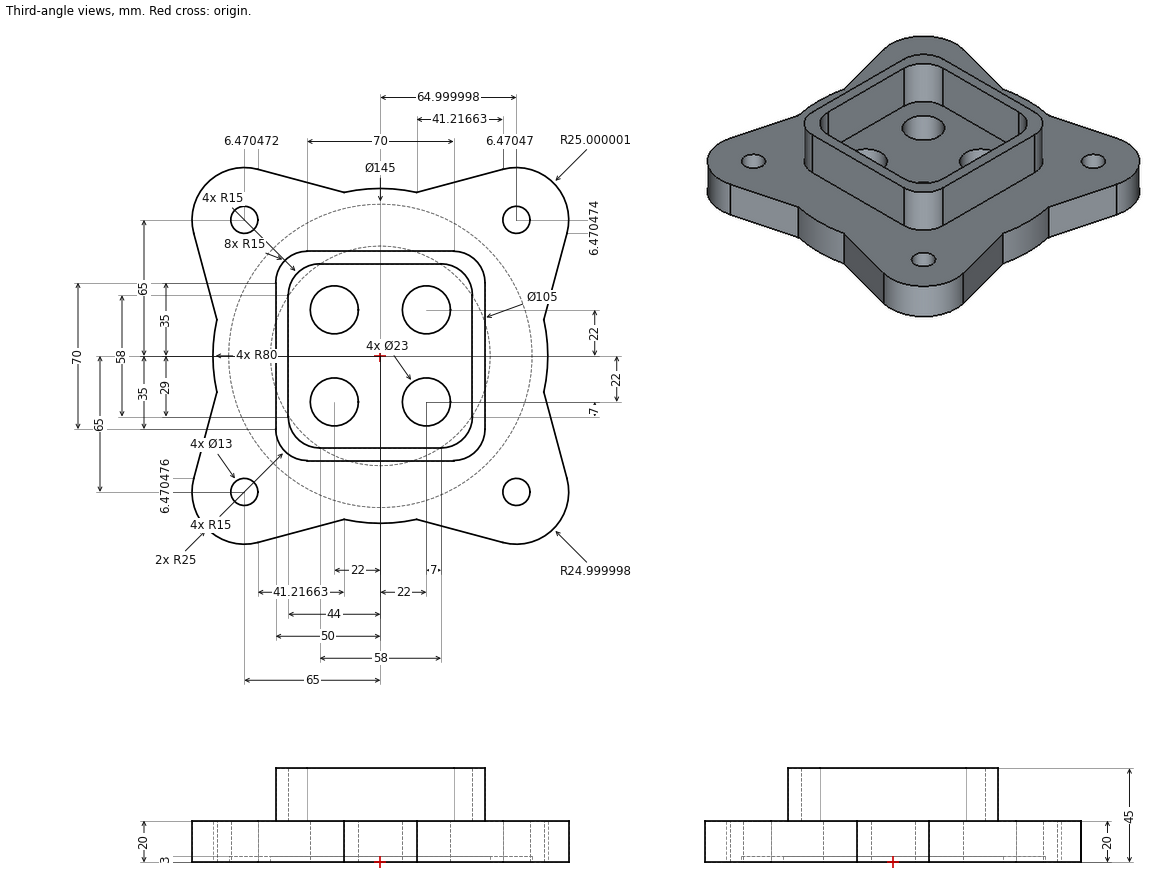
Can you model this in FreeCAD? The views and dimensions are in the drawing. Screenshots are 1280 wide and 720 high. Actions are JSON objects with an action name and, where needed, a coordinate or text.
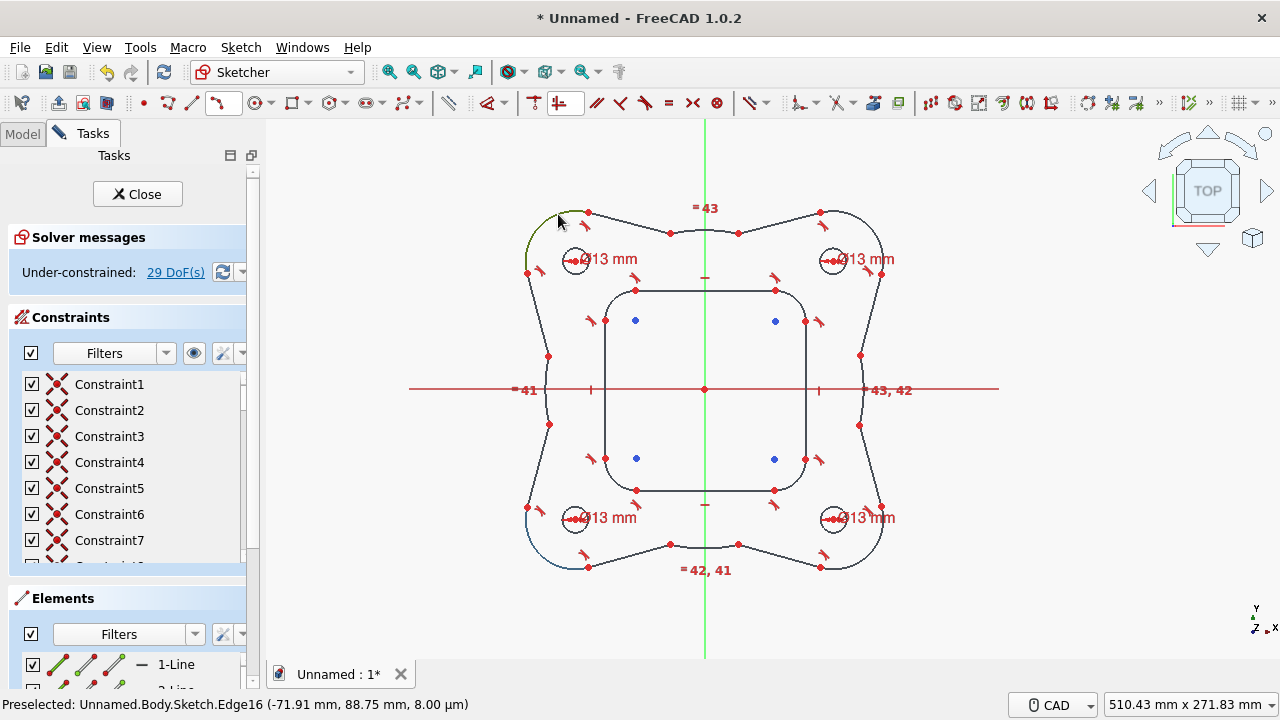
{"action": "left_click", "coordinate": [670, 104]}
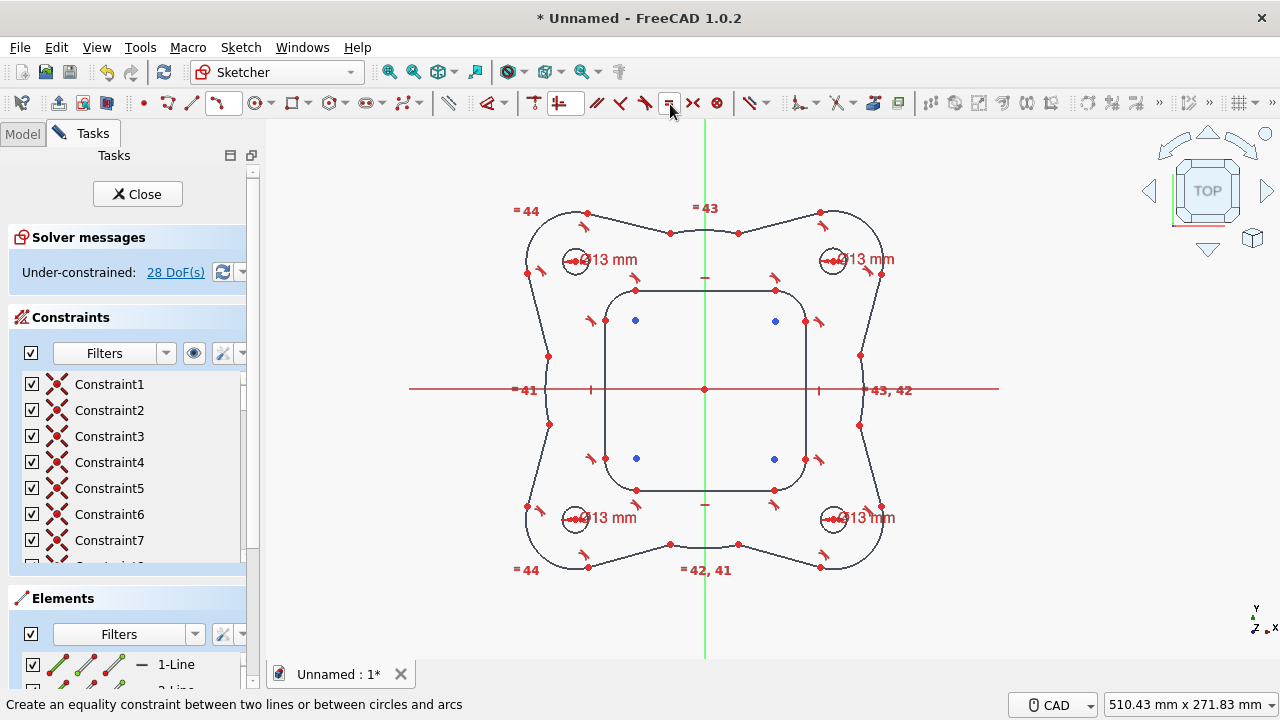
{"action": "left_click", "coordinate": [621, 294]}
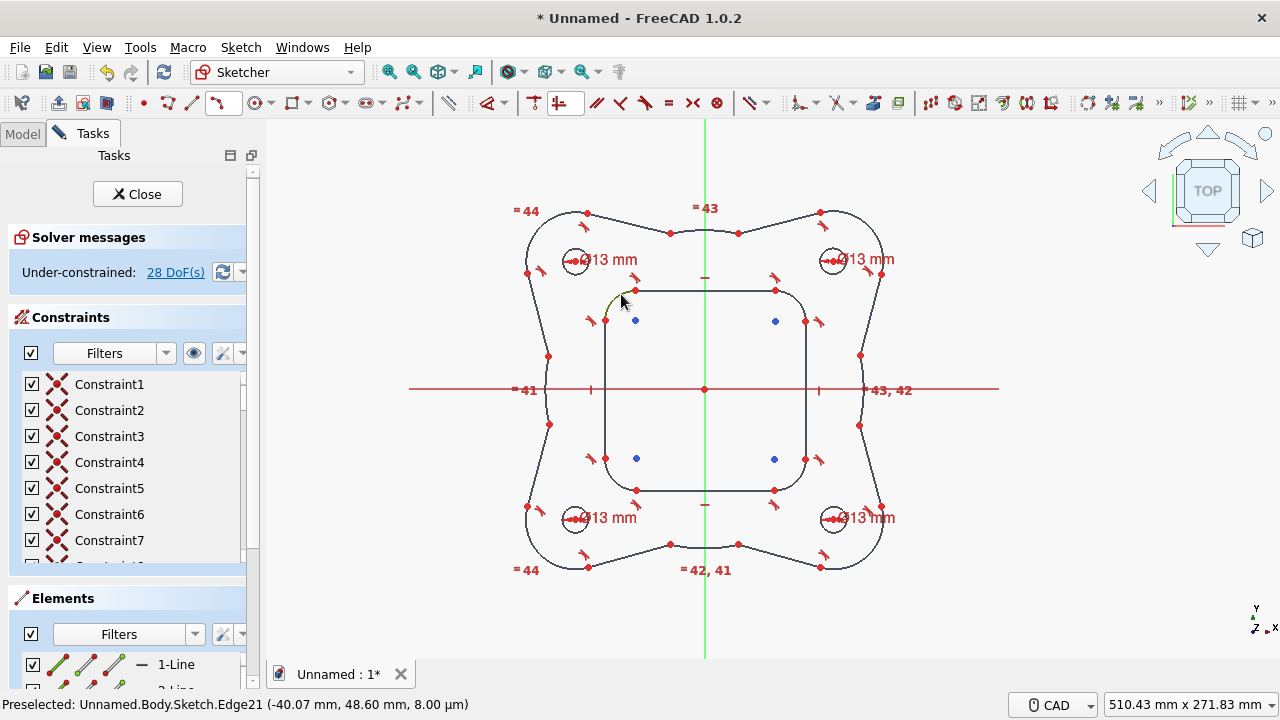
{"action": "left_click", "coordinate": [802, 308]}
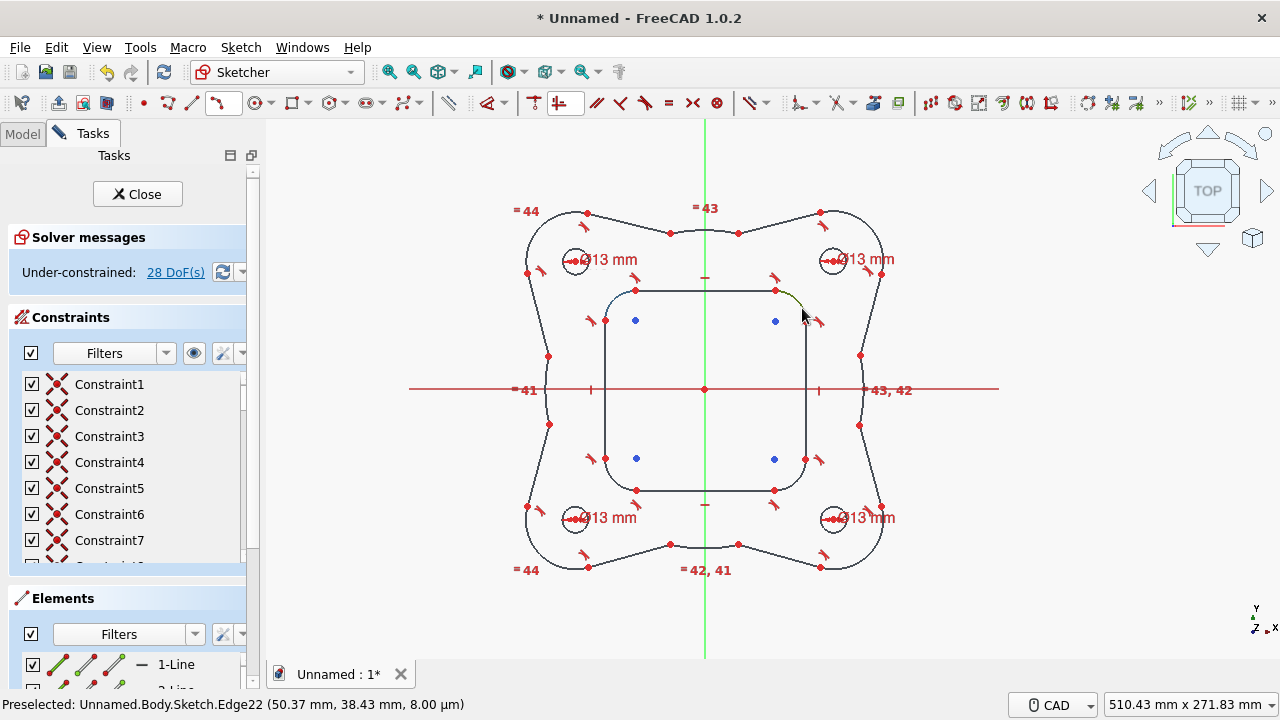
{"action": "left_click", "coordinate": [789, 487]}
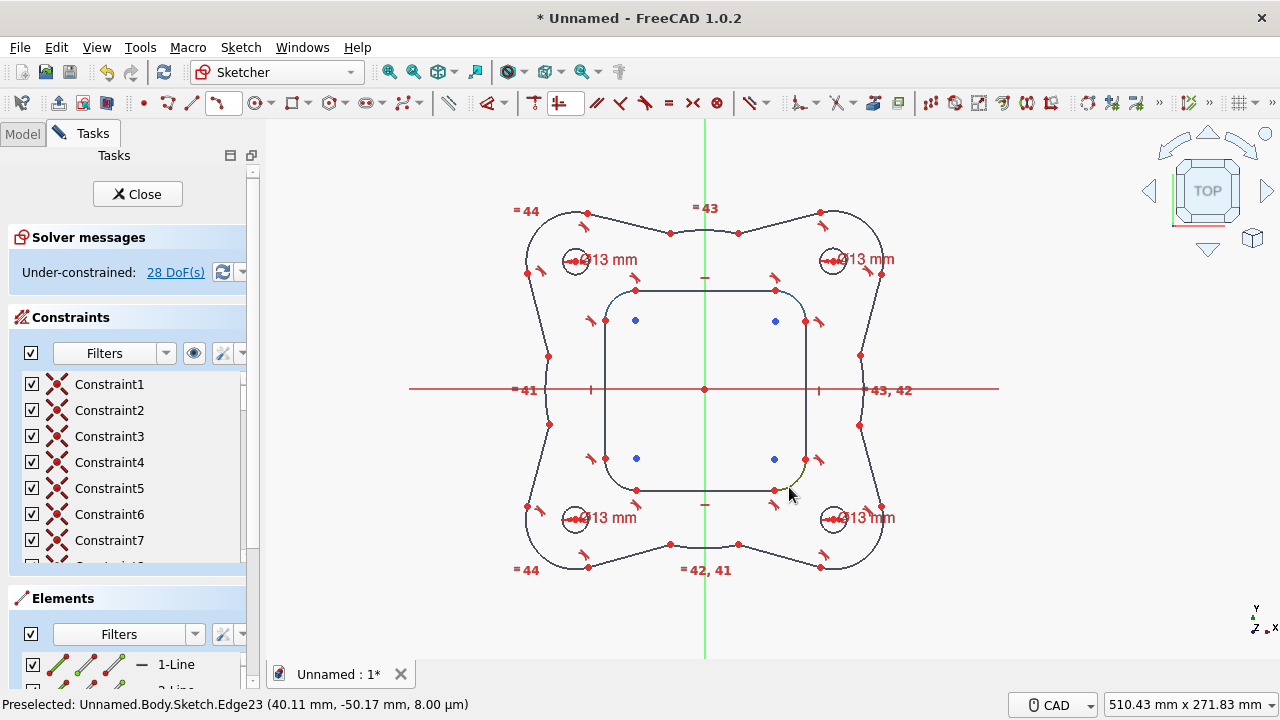
{"action": "left_click", "coordinate": [609, 473]}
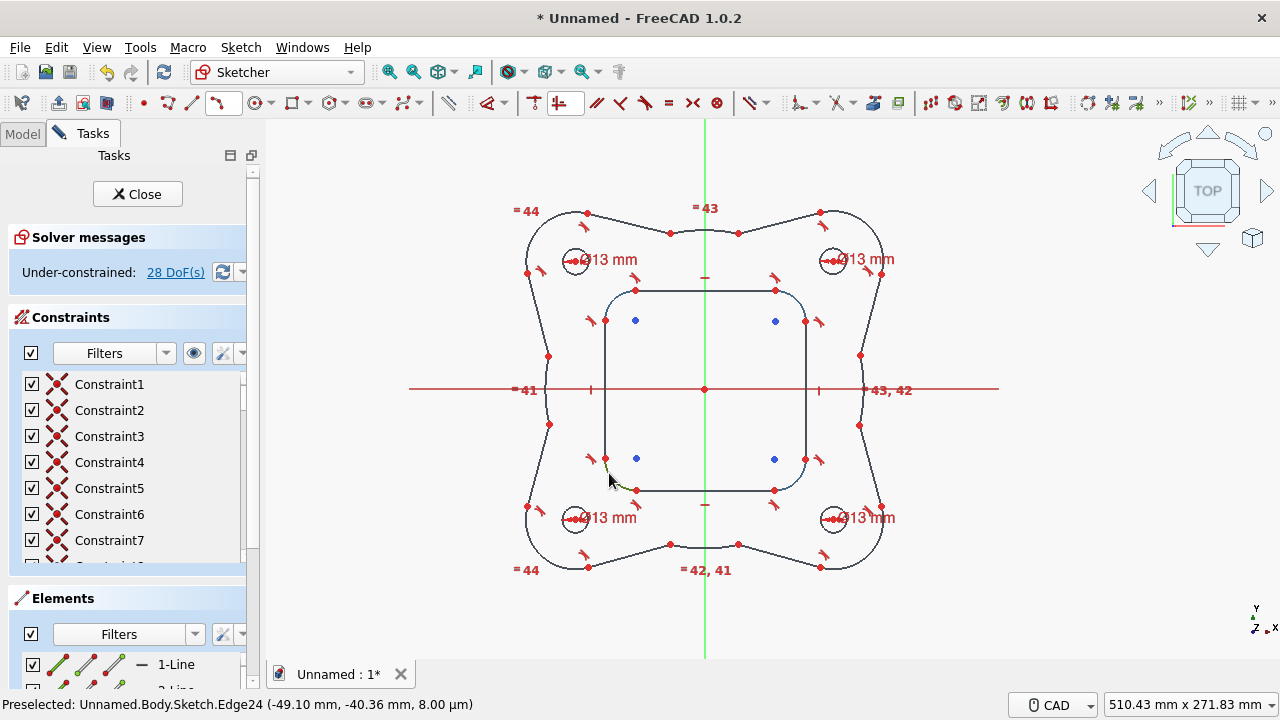
{"action": "left_click", "coordinate": [670, 104]}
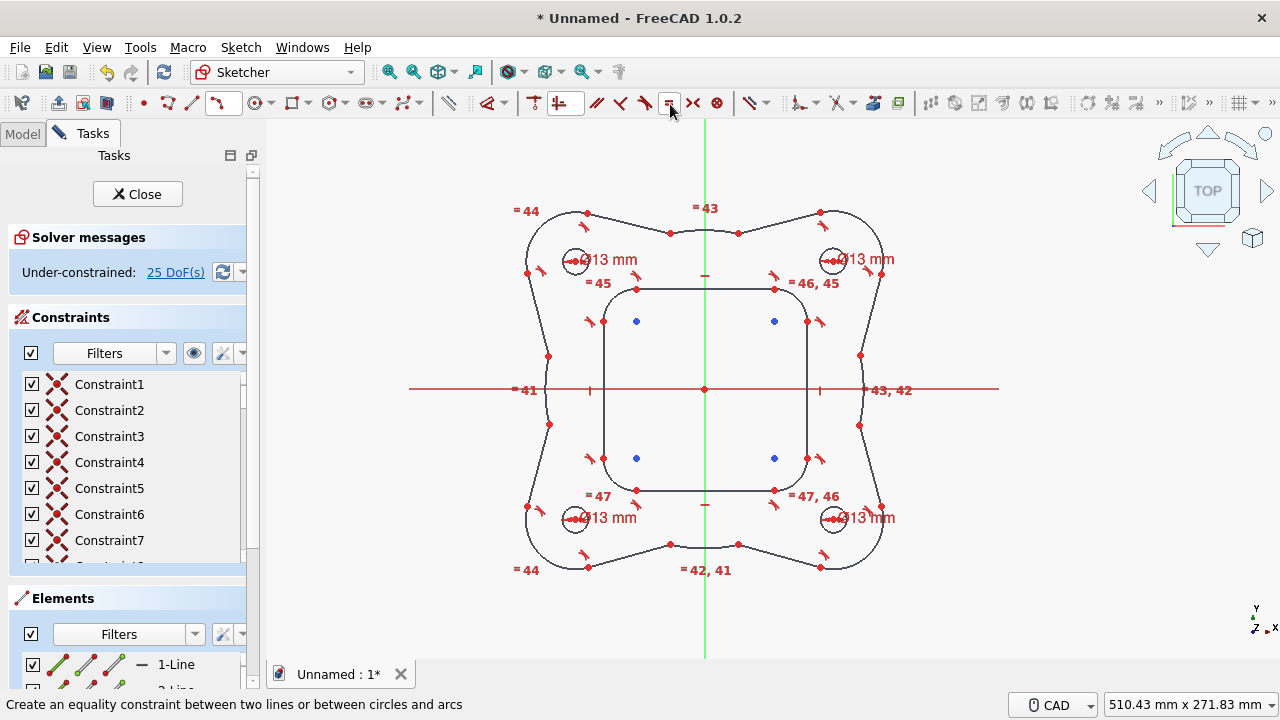
{"action": "left_click", "coordinate": [488, 104]}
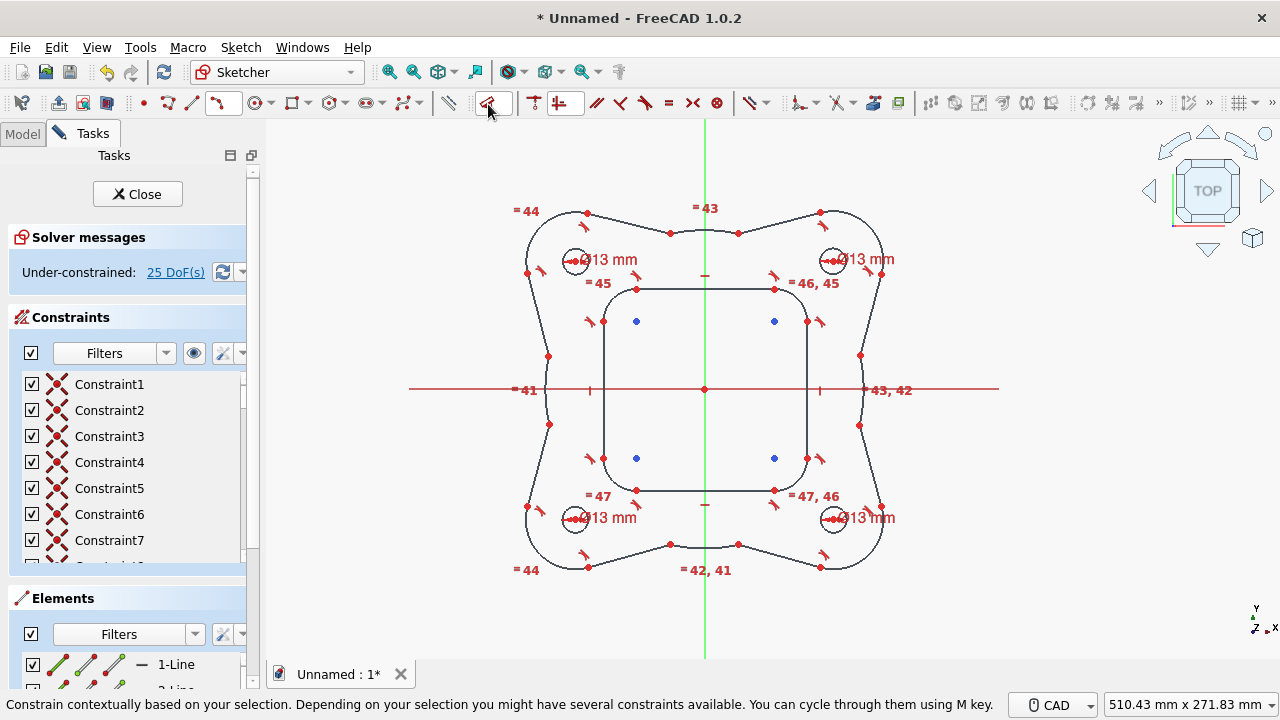
{"action": "left_click", "coordinate": [546, 377]}
{"action": "left_click", "coordinate": [514, 375]}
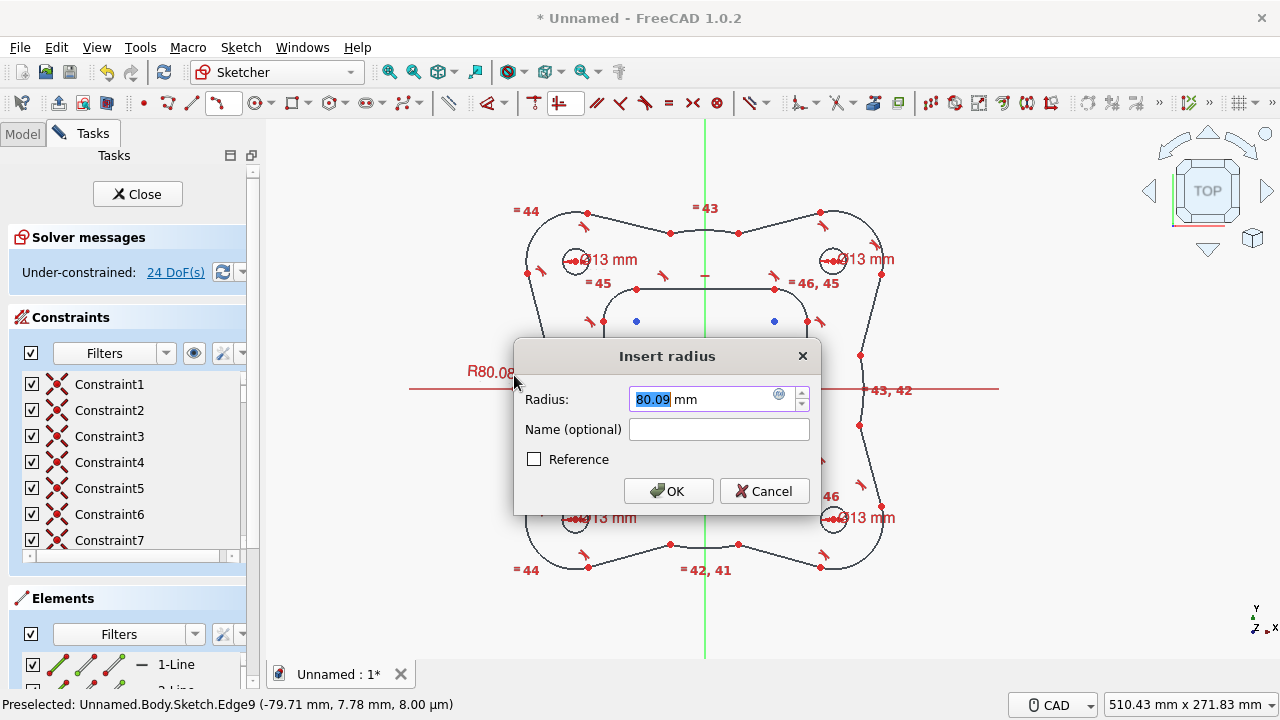
{"action": "type", "text": "80"}
{"action": "key", "text": "Return"}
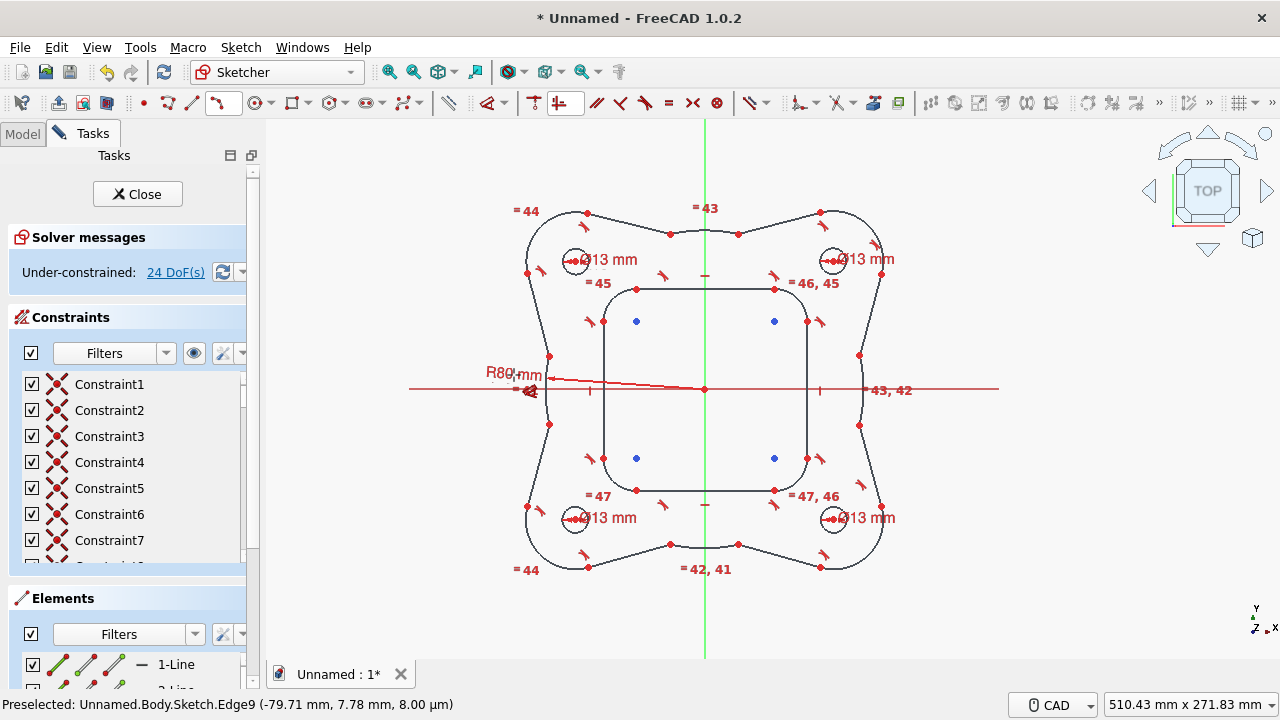
{"action": "left_click", "coordinate": [529, 538]}
{"action": "left_click", "coordinate": [499, 550]}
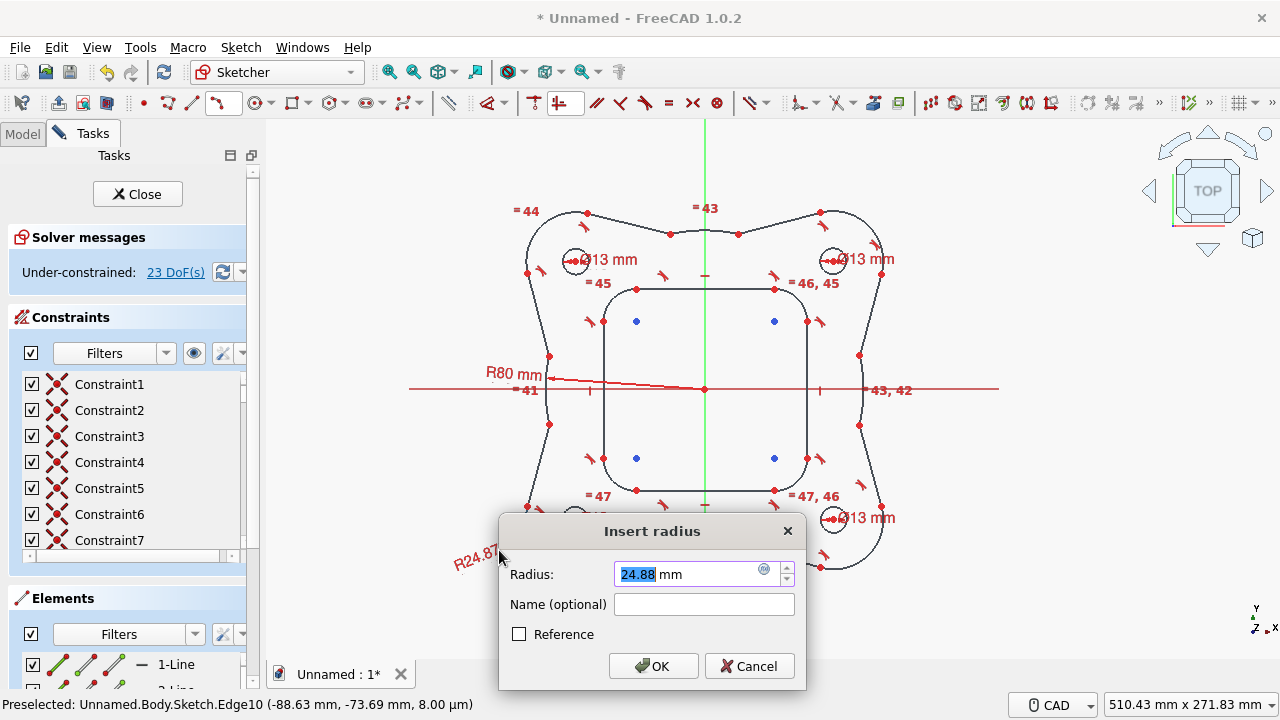
{"action": "type", "text": "25"}
{"action": "key", "text": "Return"}